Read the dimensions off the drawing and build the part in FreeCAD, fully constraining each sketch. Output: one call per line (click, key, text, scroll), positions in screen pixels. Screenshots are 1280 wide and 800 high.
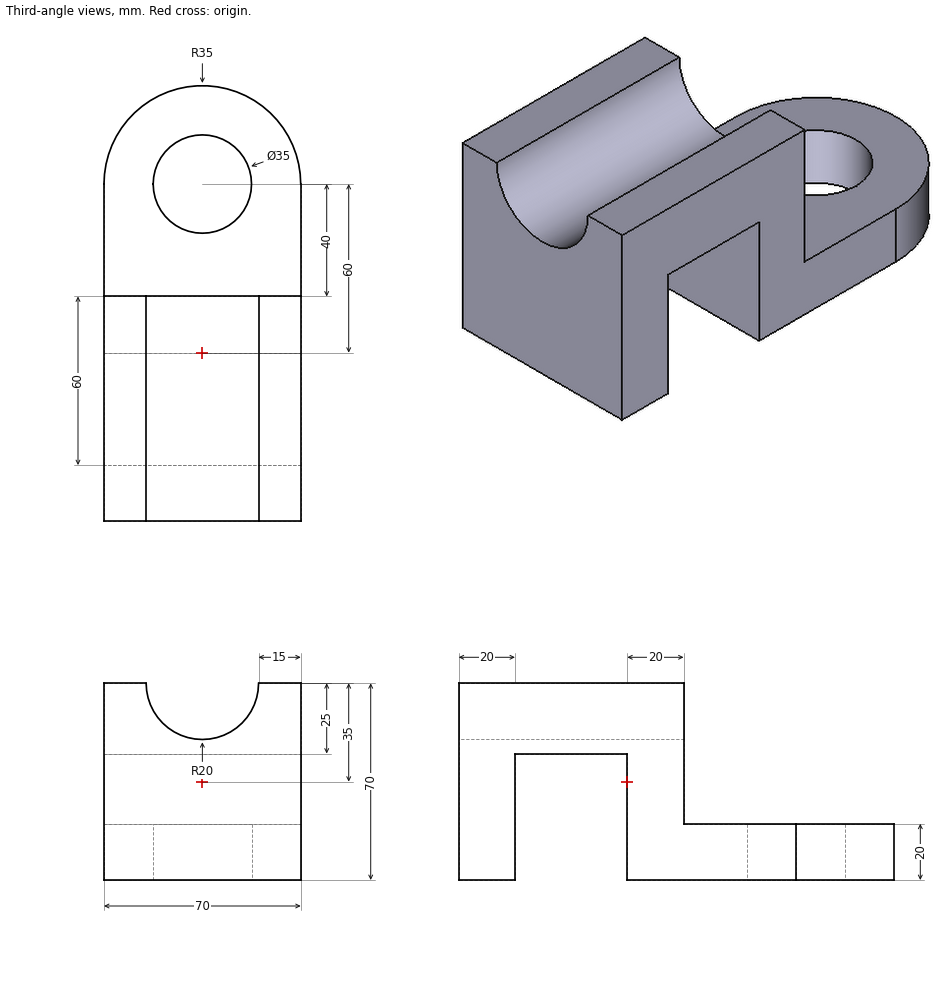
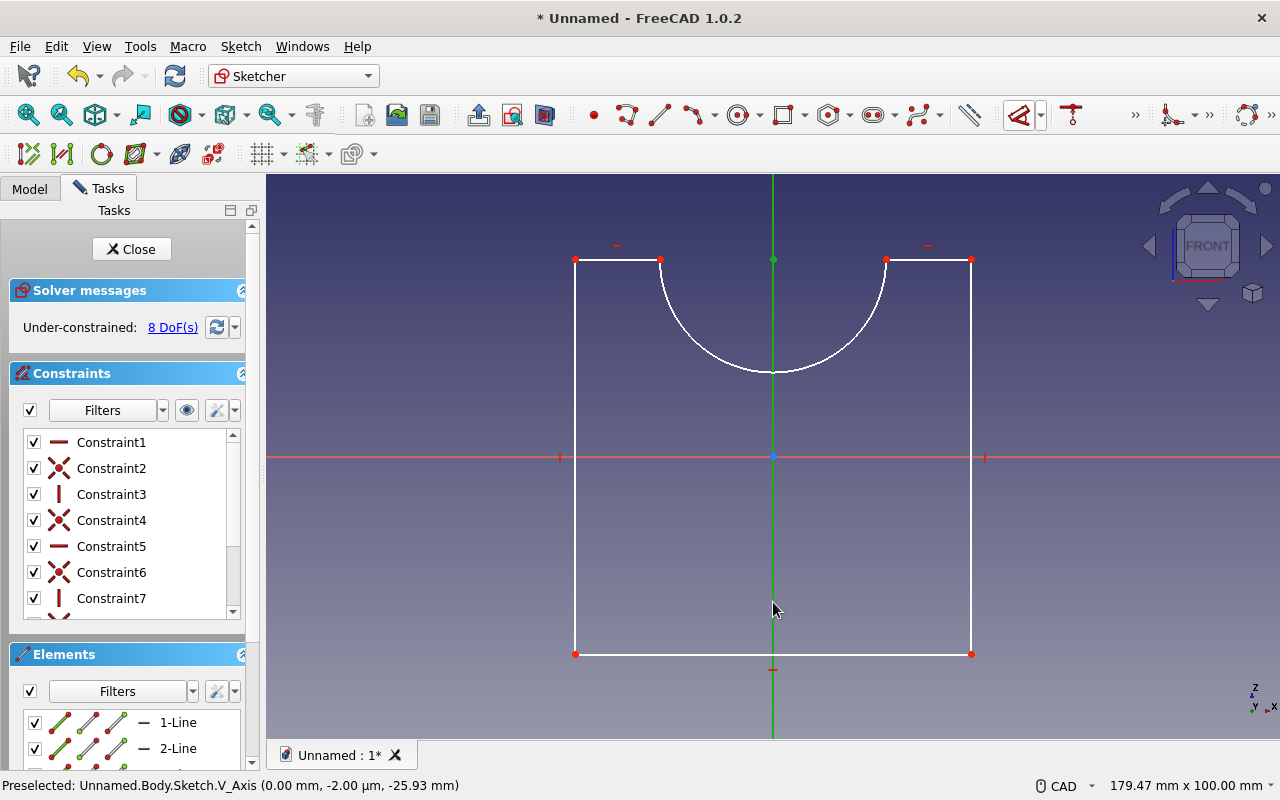
click(1071, 116)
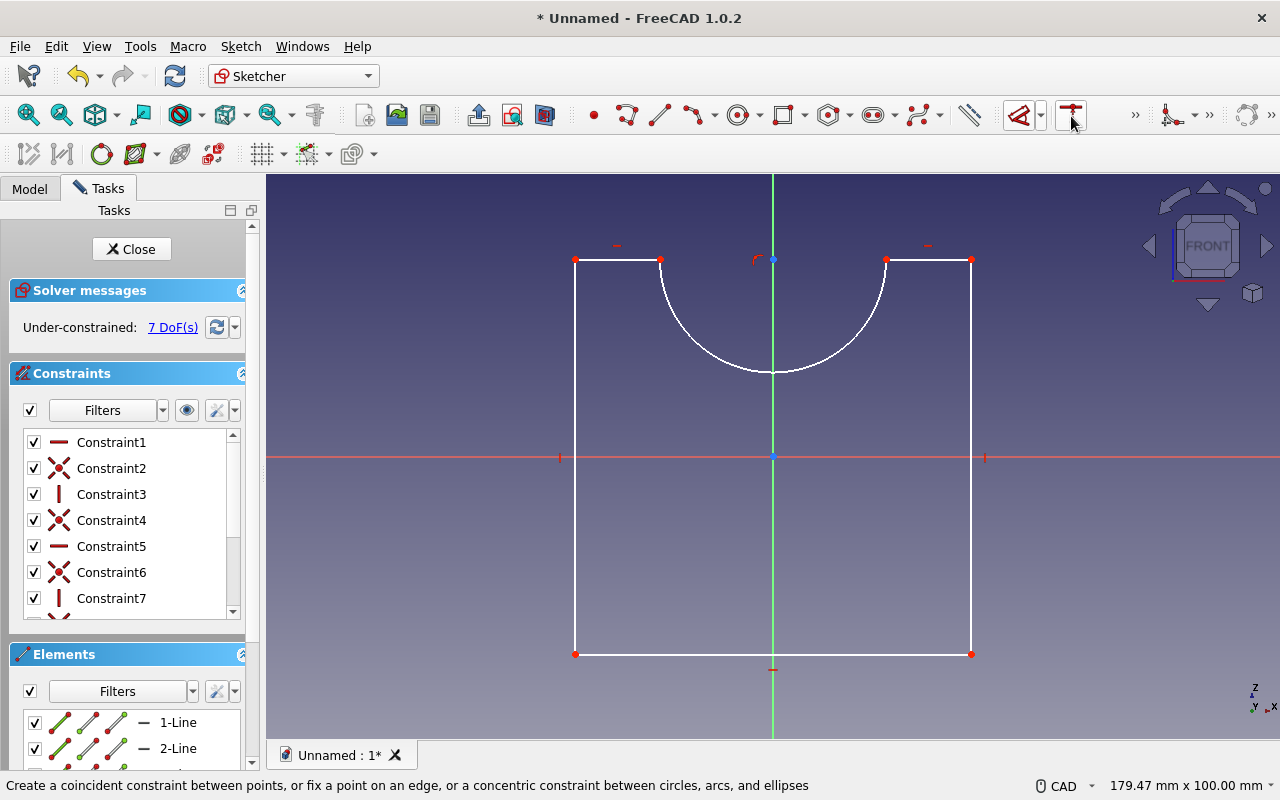
click(1018, 116)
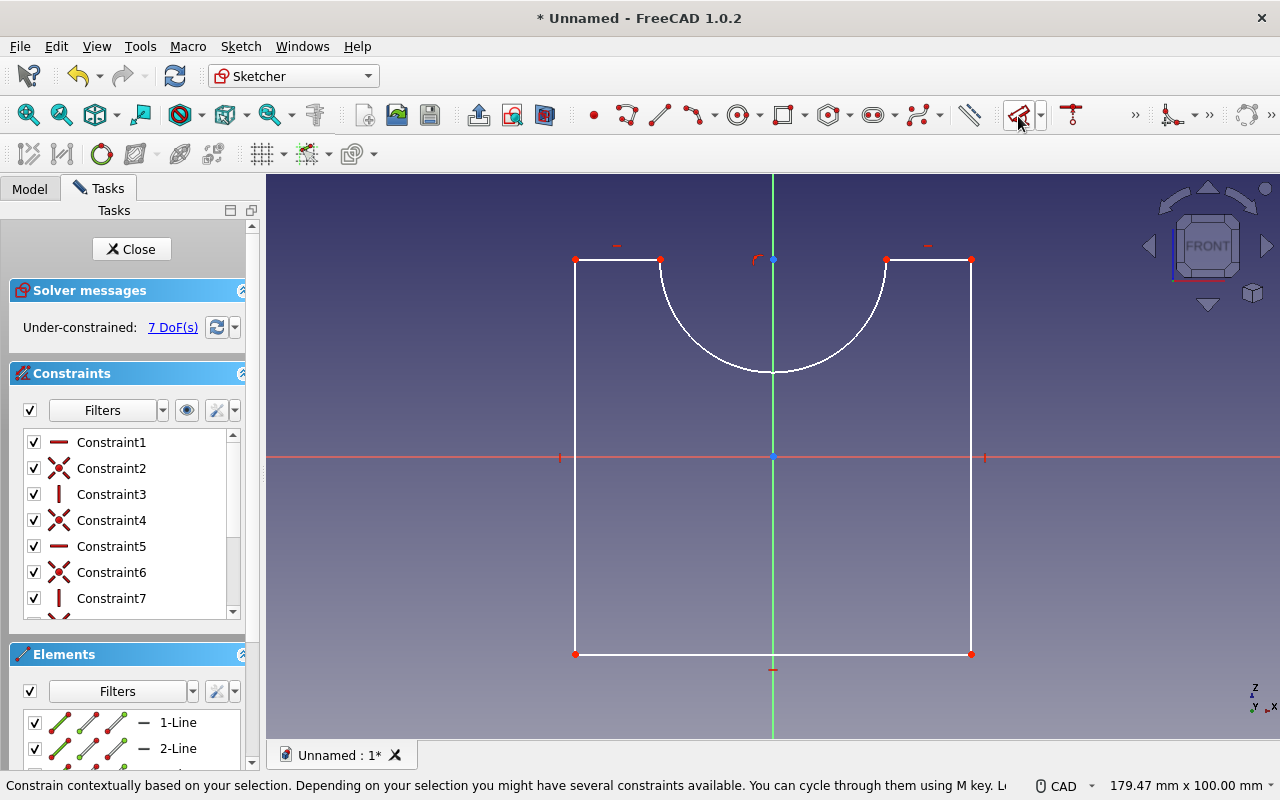
click(707, 351)
click(688, 377)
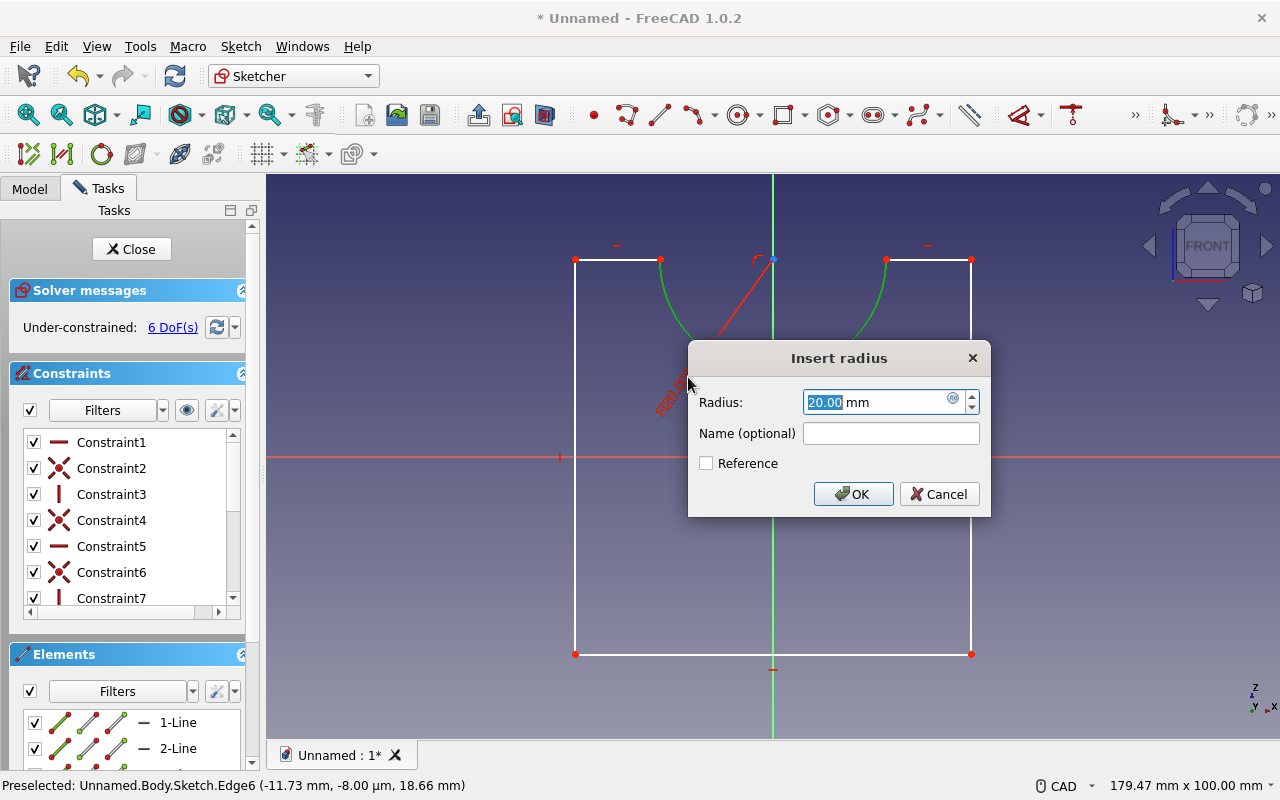
text(20)
key(Return)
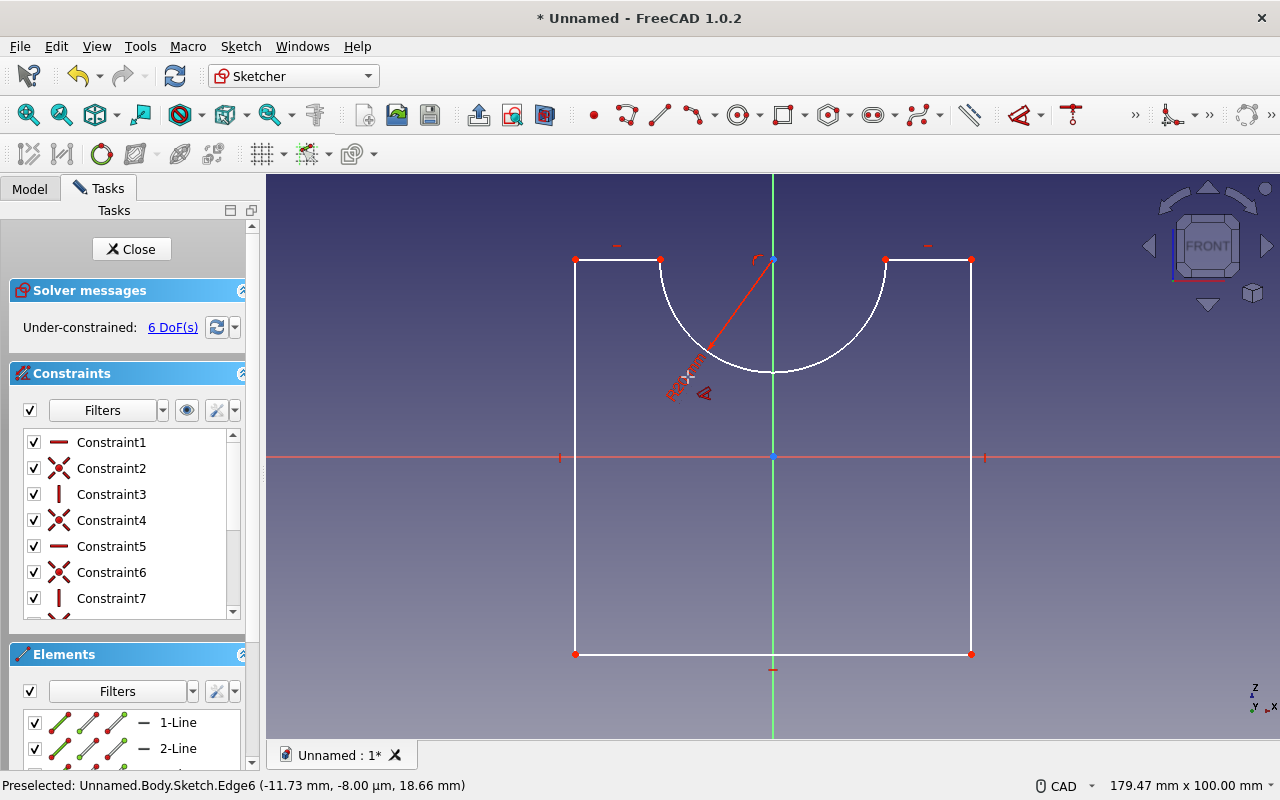
click(911, 260)
click(928, 226)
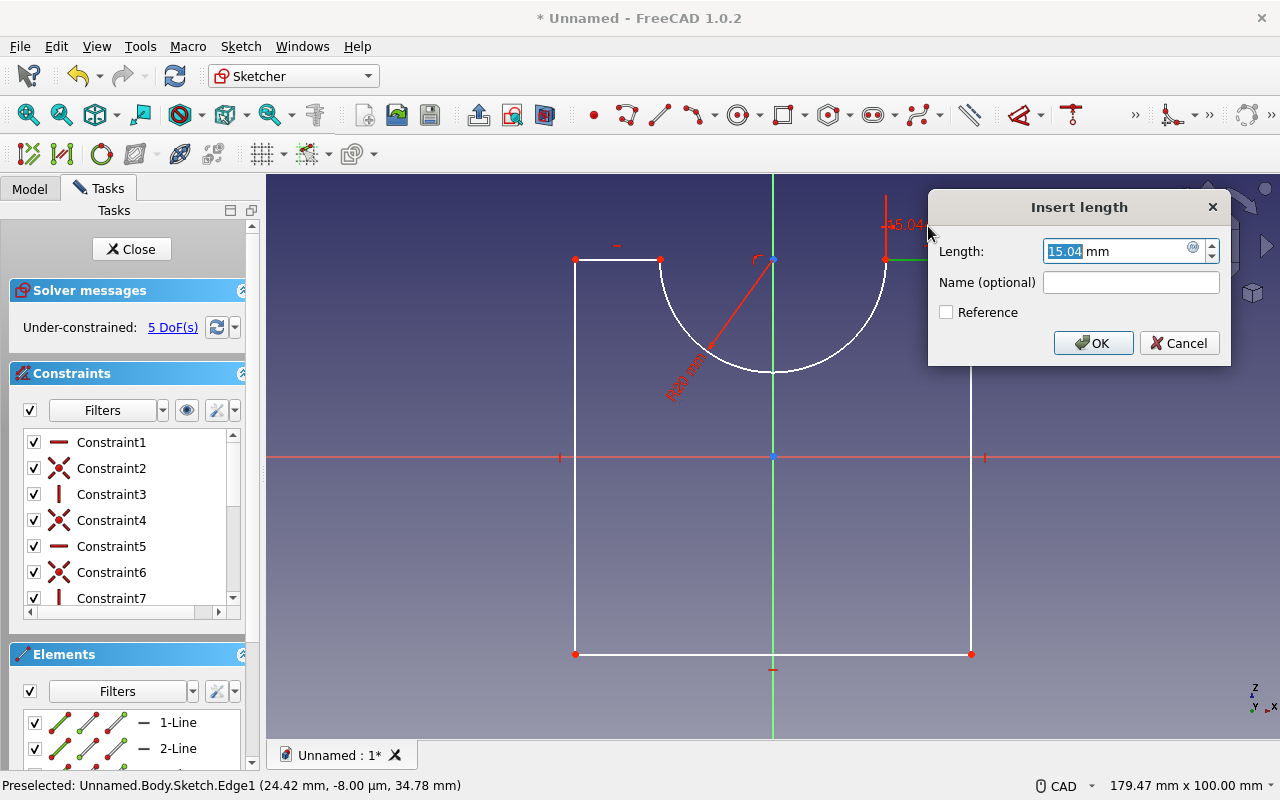
text(15)
key(Return)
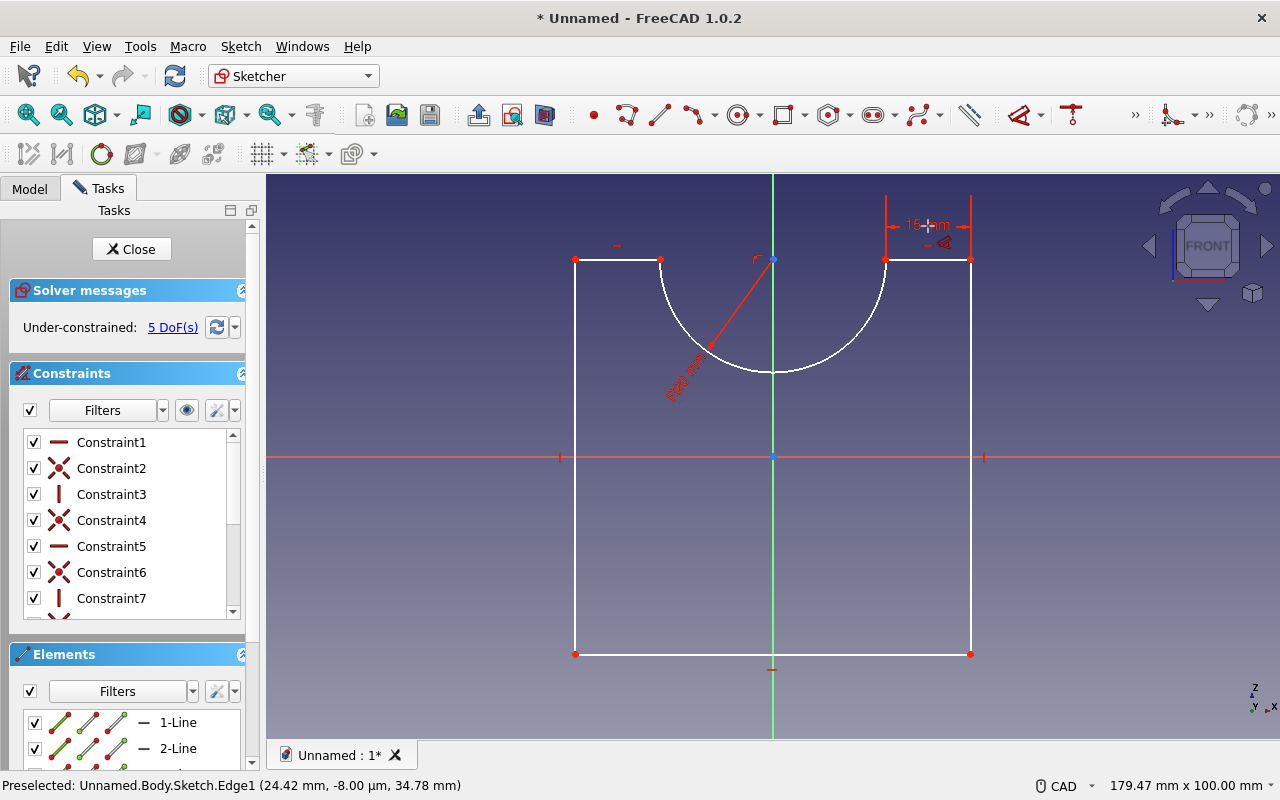
click(971, 378)
click(1005, 367)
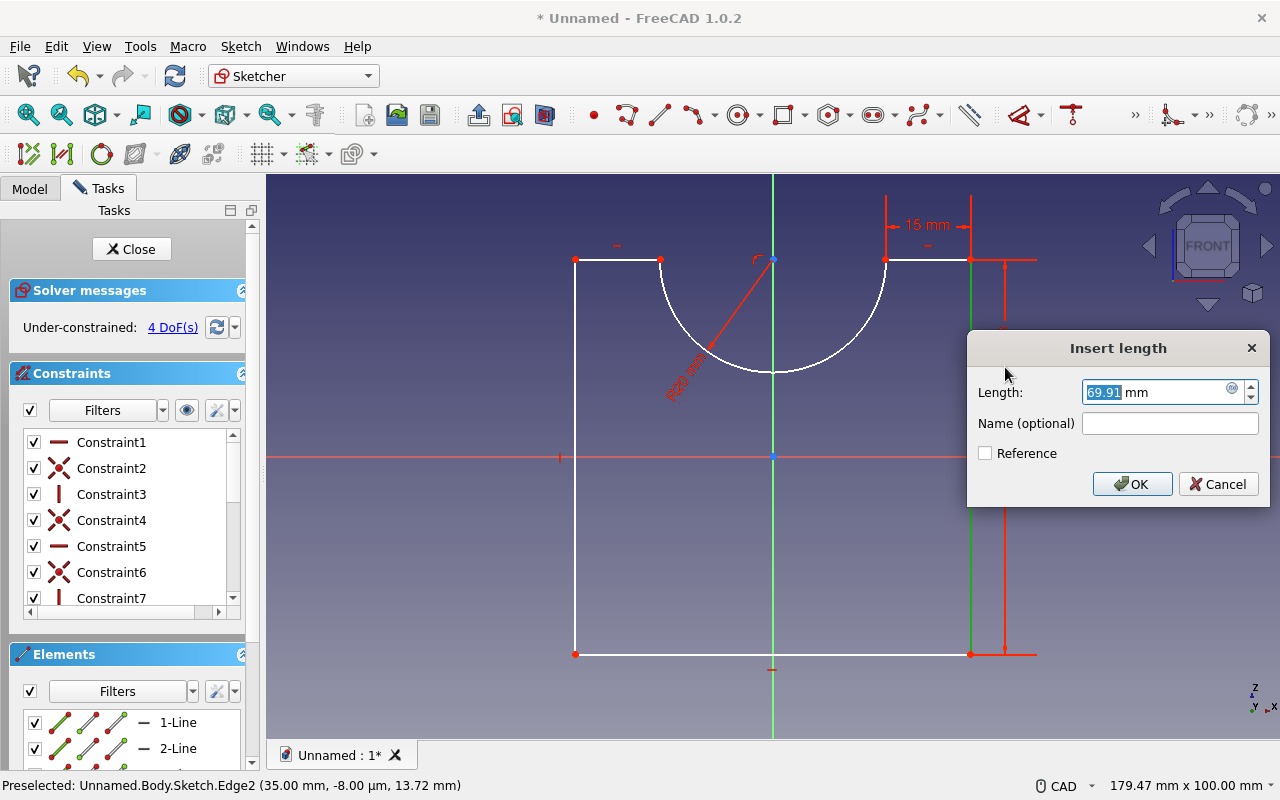
text(70)
key(Return)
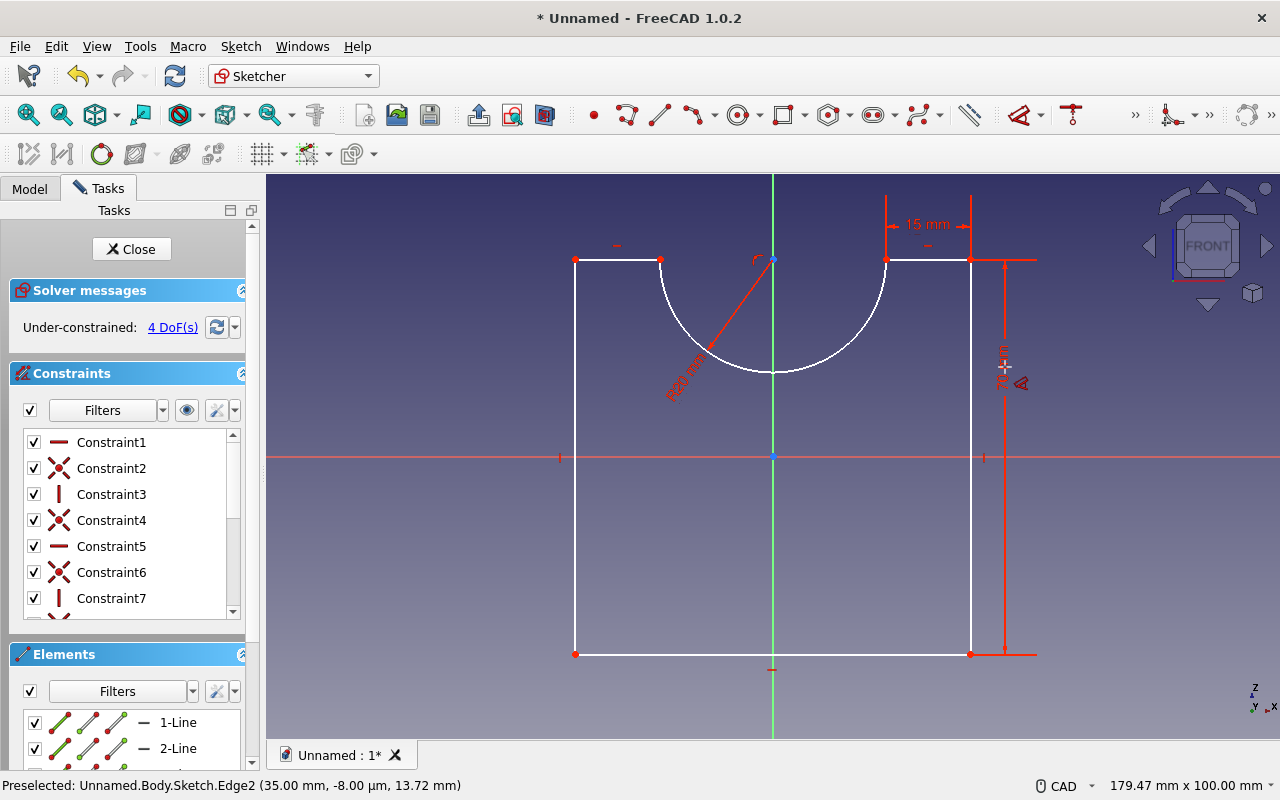
click(852, 655)
click(682, 689)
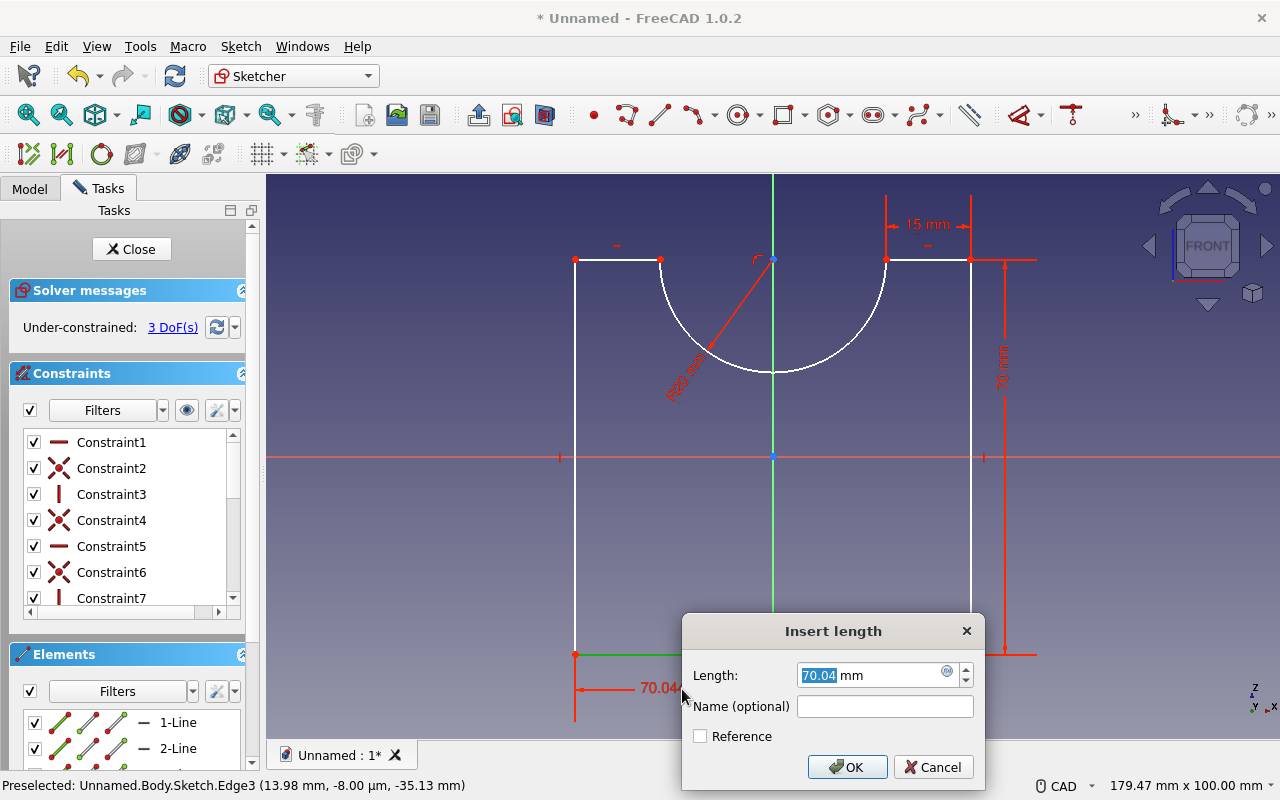
text(70)
key(Return)